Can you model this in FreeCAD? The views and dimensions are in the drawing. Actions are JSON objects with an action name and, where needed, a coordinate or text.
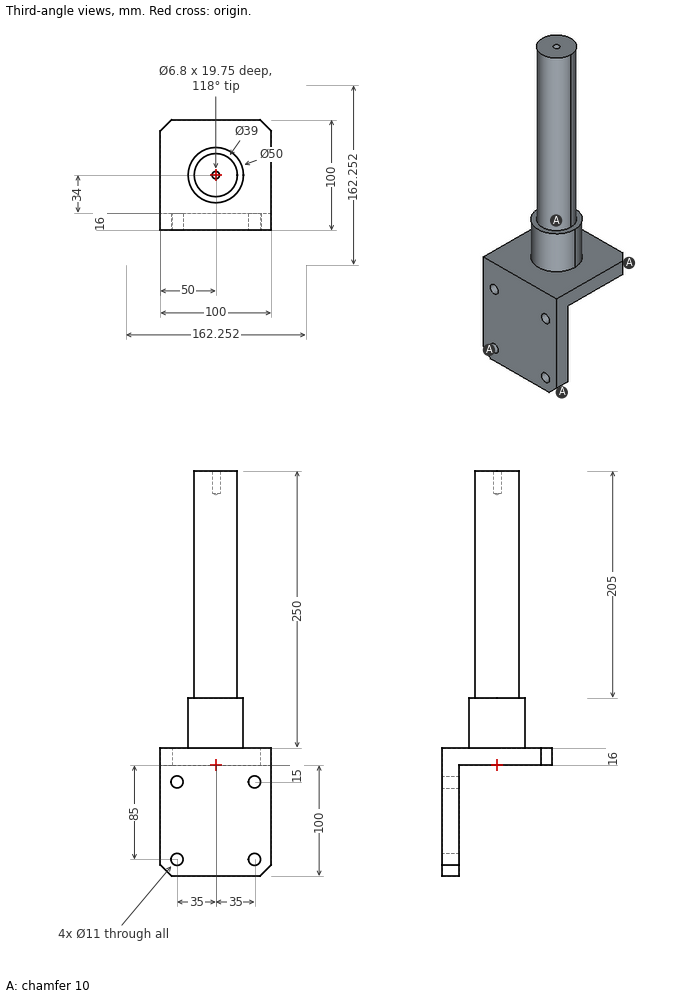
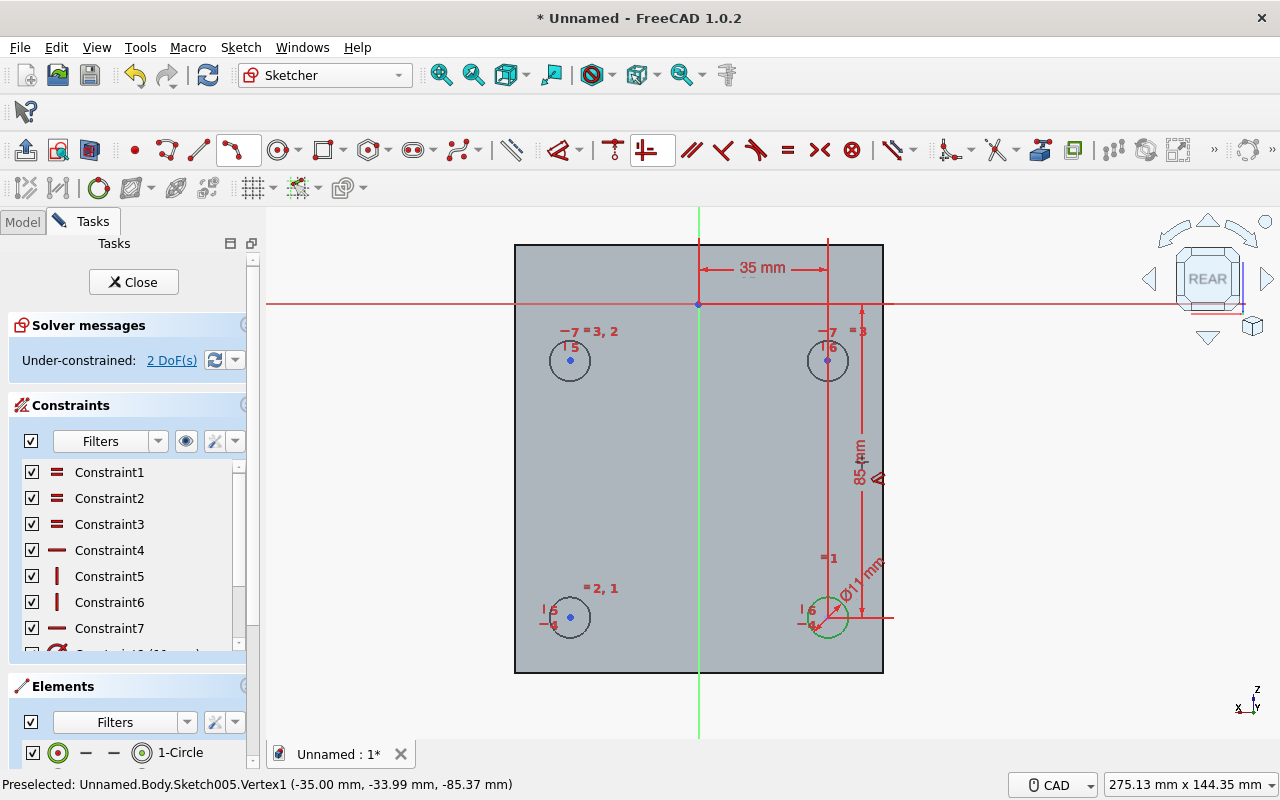
{"action": "left_click", "coordinate": [570, 618]}
{"action": "left_click", "coordinate": [634, 270]}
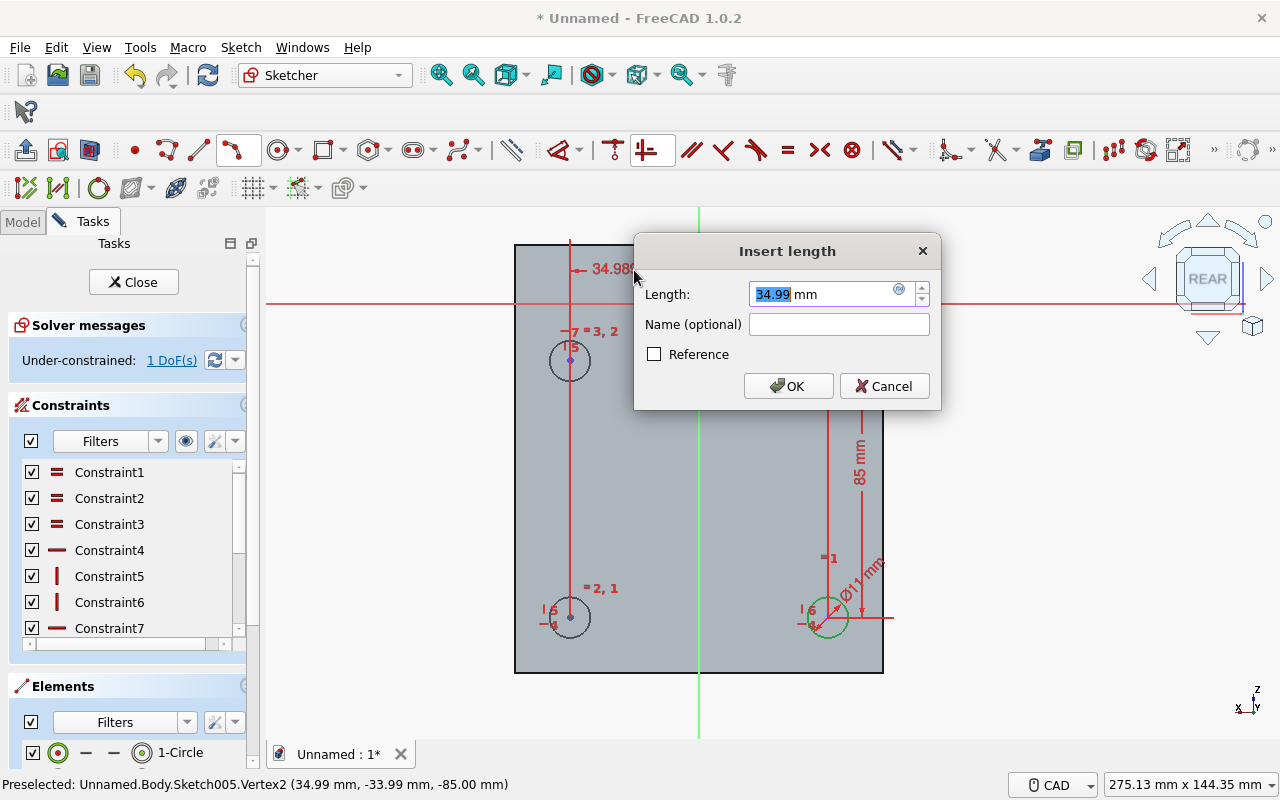
{"action": "type", "text": "35"}
{"action": "key", "text": "Return"}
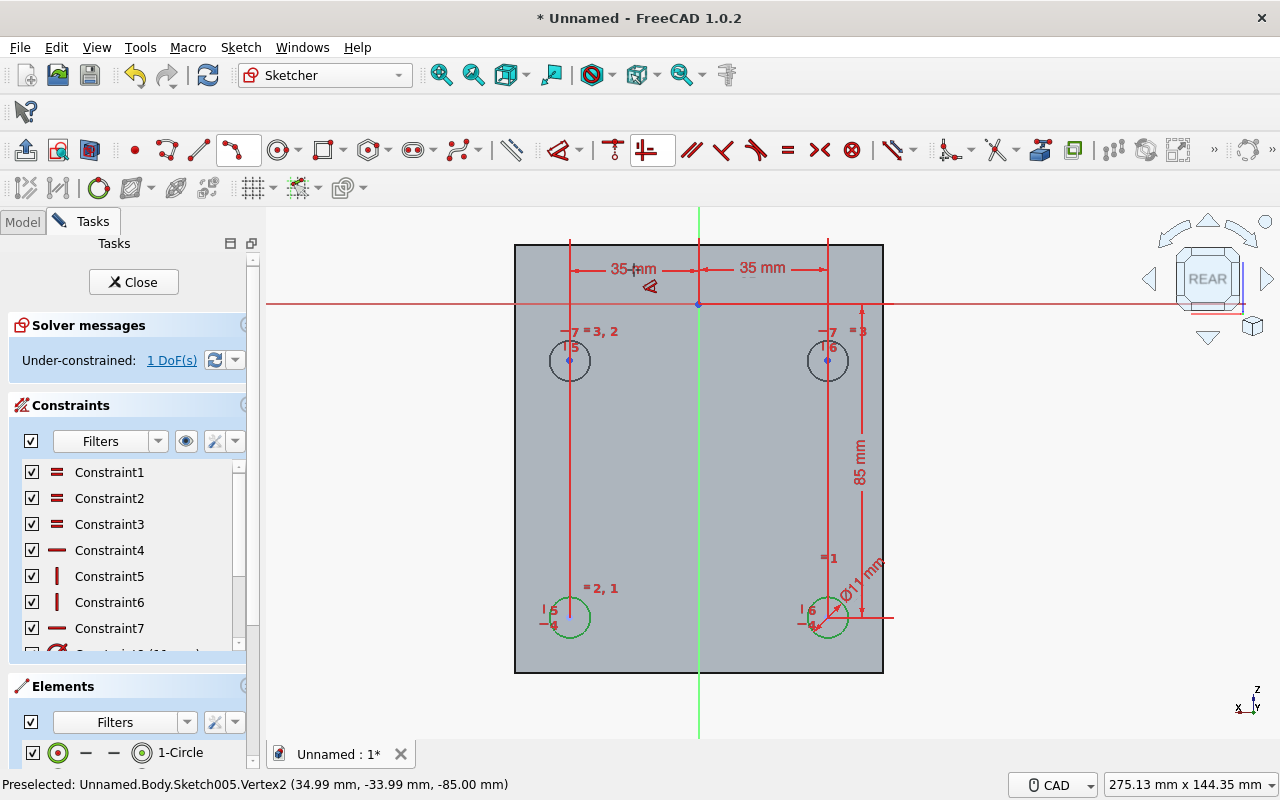
{"action": "left_click", "coordinate": [570, 361]}
{"action": "left_click", "coordinate": [536, 333]}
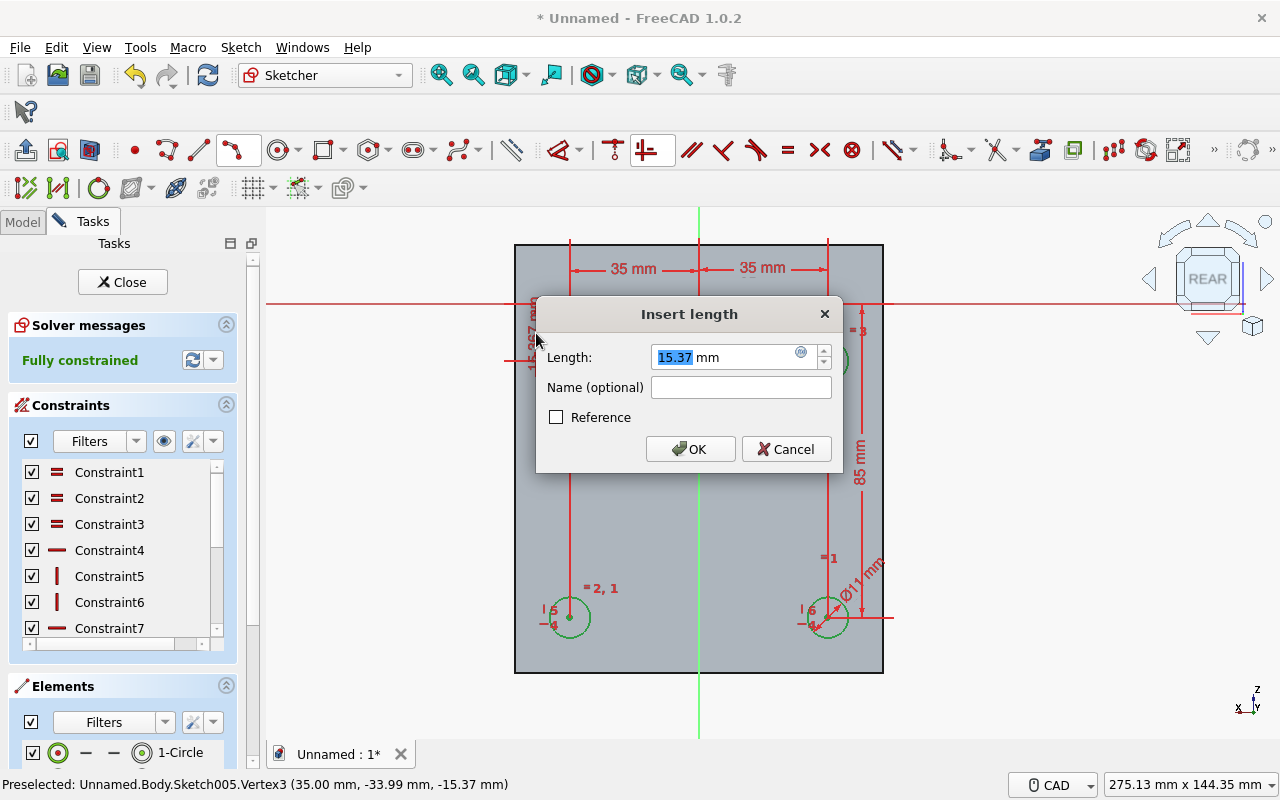
{"action": "type", "text": "15"}
{"action": "key", "text": "Return"}
{"action": "key", "text": "Escape"}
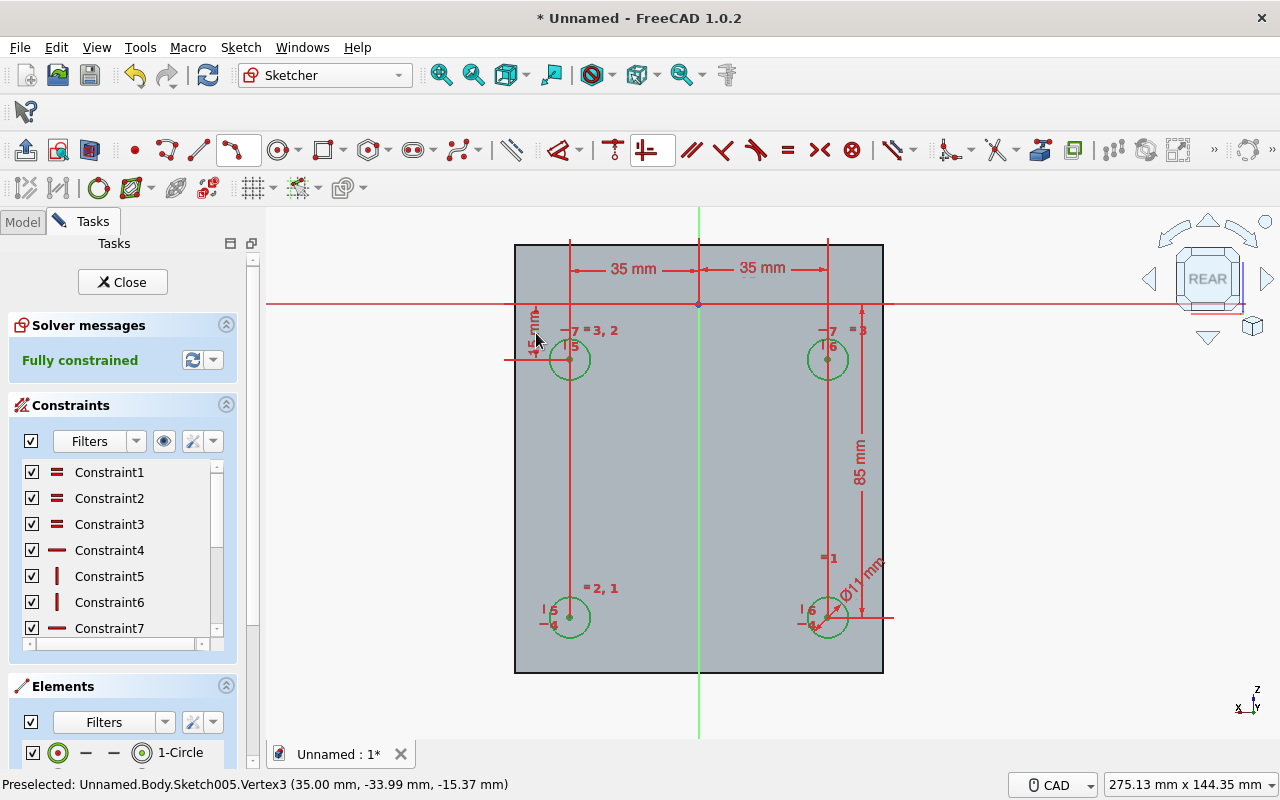
{"action": "left_click", "coordinate": [123, 282]}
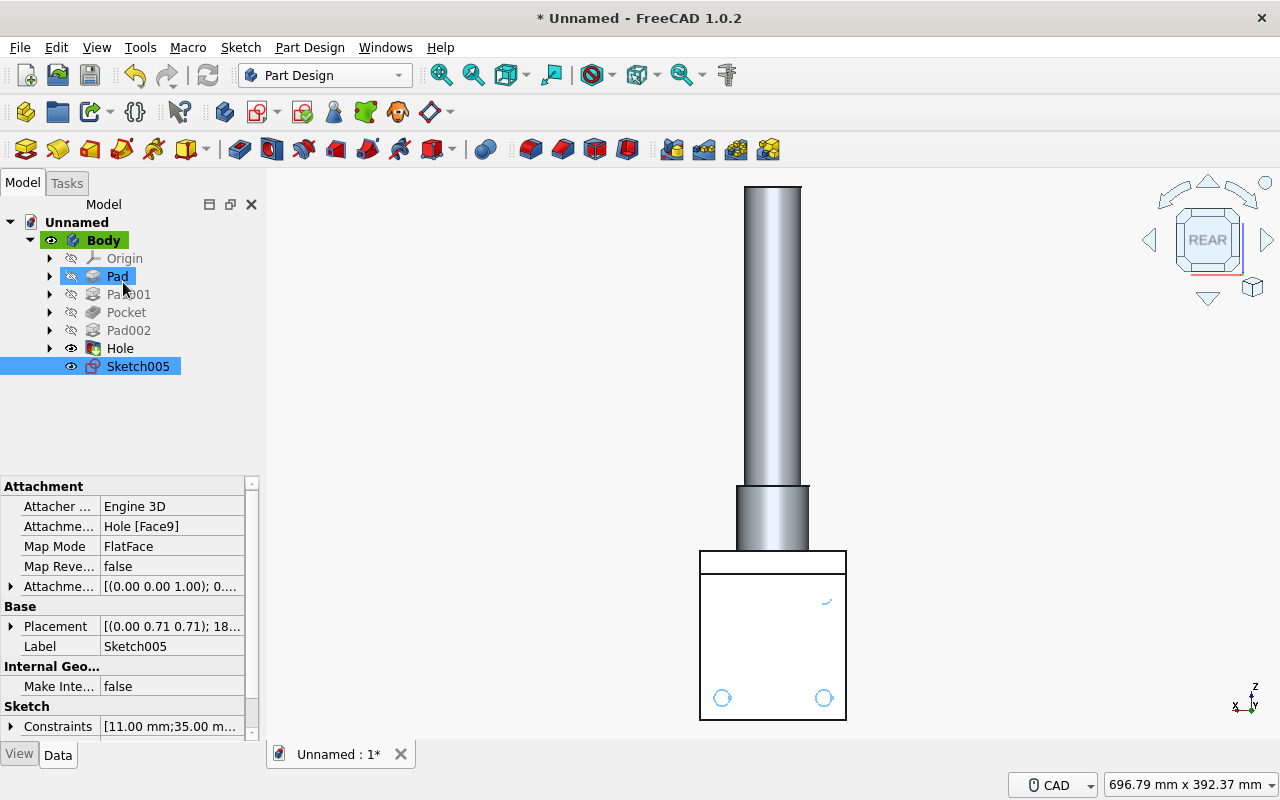
{"action": "left_click", "coordinate": [272, 150]}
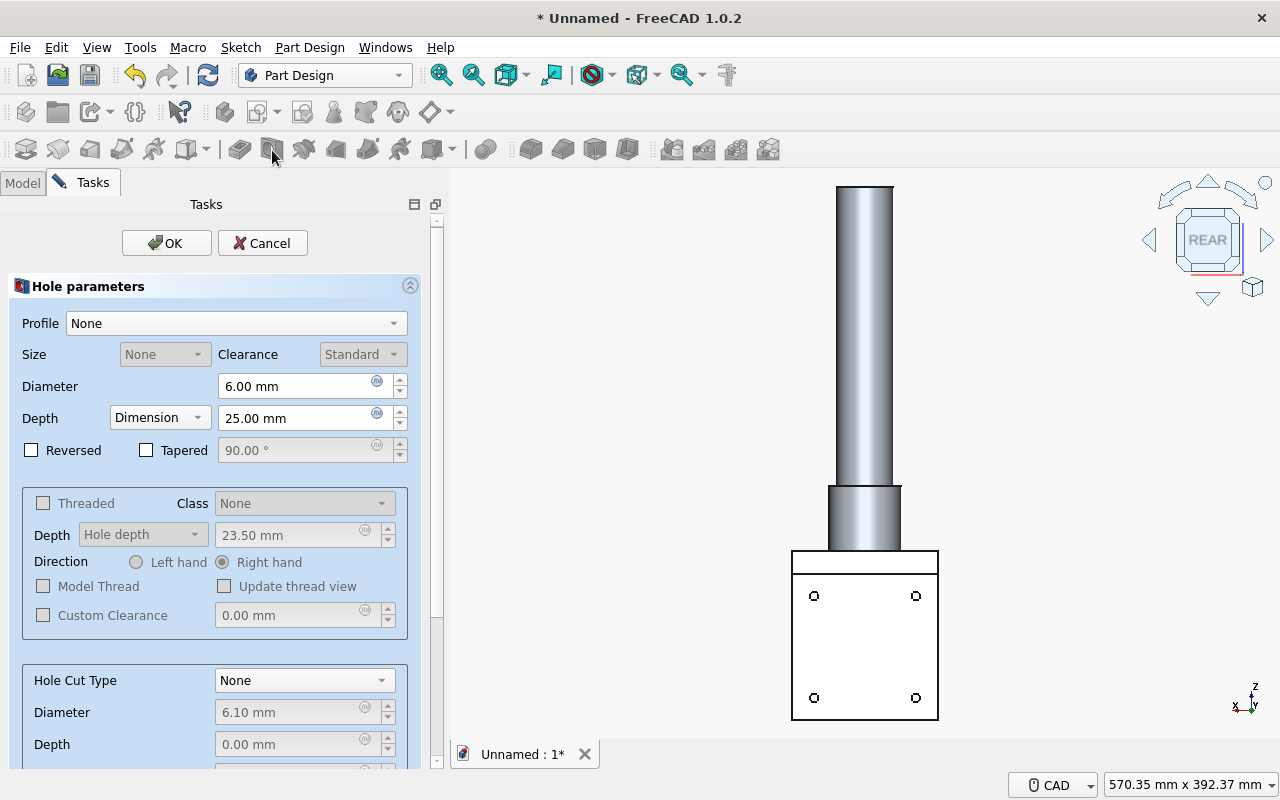
{"action": "triple_click", "coordinate": [305, 386]}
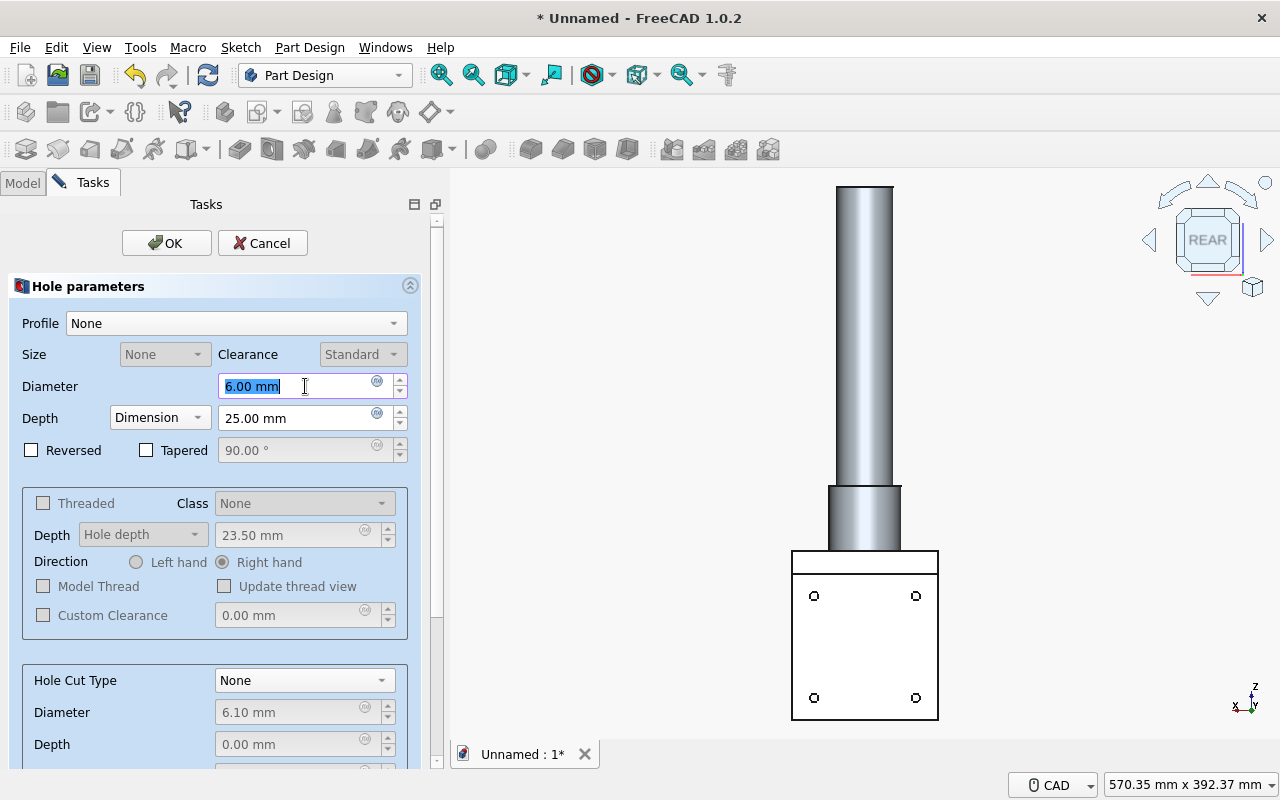
{"action": "type", "text": "11"}
{"action": "key", "text": "Tab"}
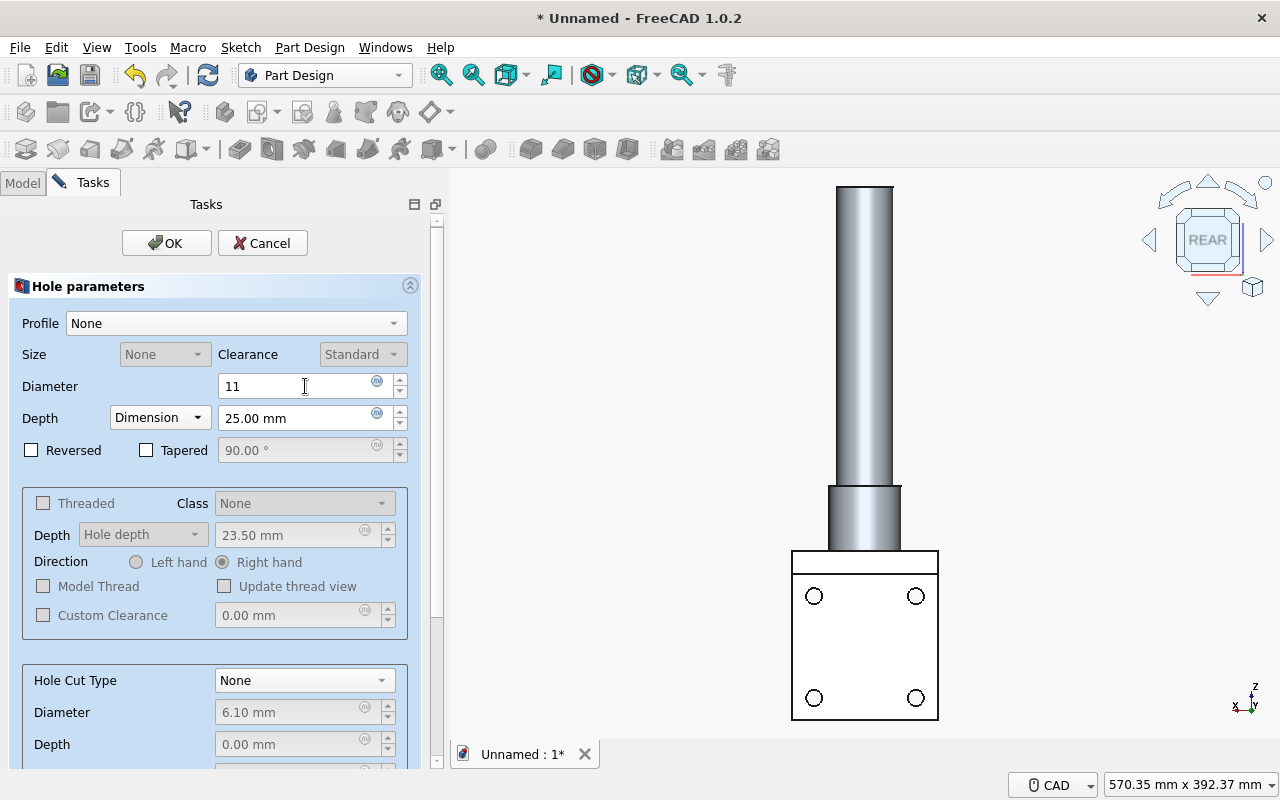
{"action": "left_click", "coordinate": [161, 418]}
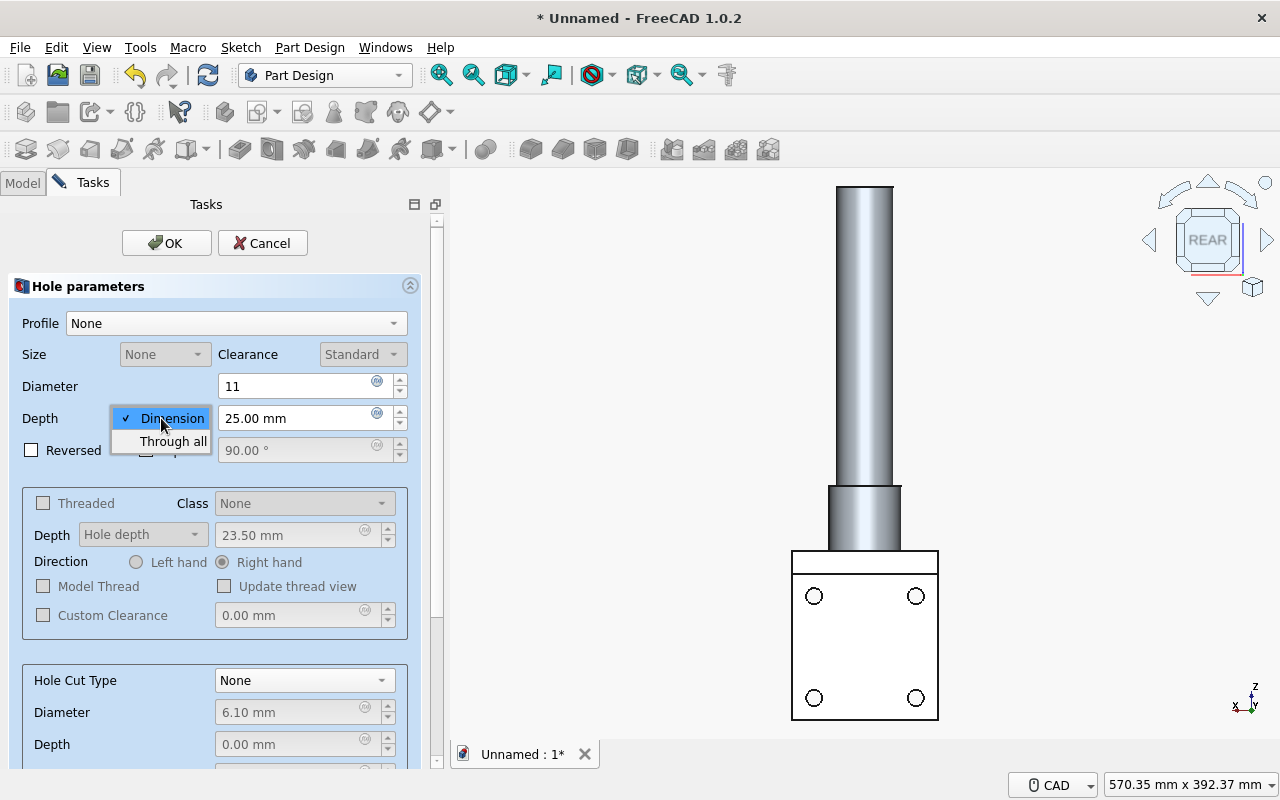
{"action": "left_click", "coordinate": [160, 442]}